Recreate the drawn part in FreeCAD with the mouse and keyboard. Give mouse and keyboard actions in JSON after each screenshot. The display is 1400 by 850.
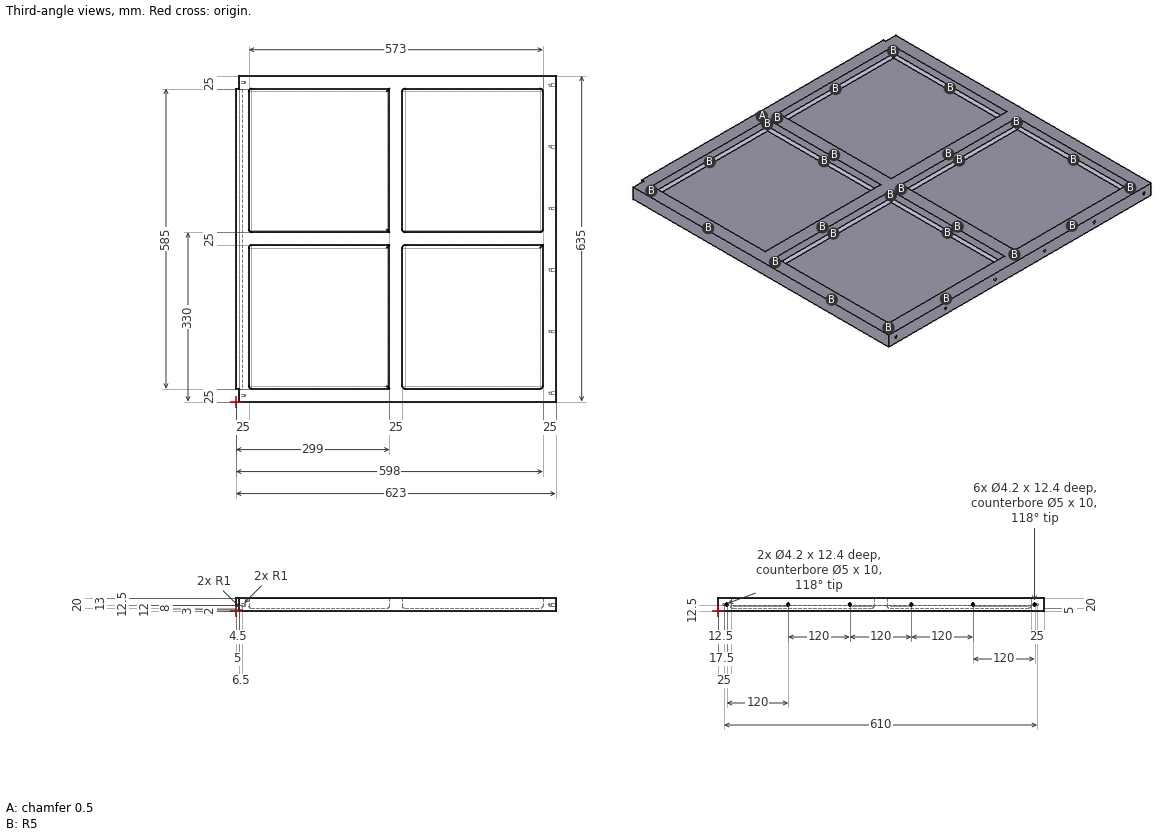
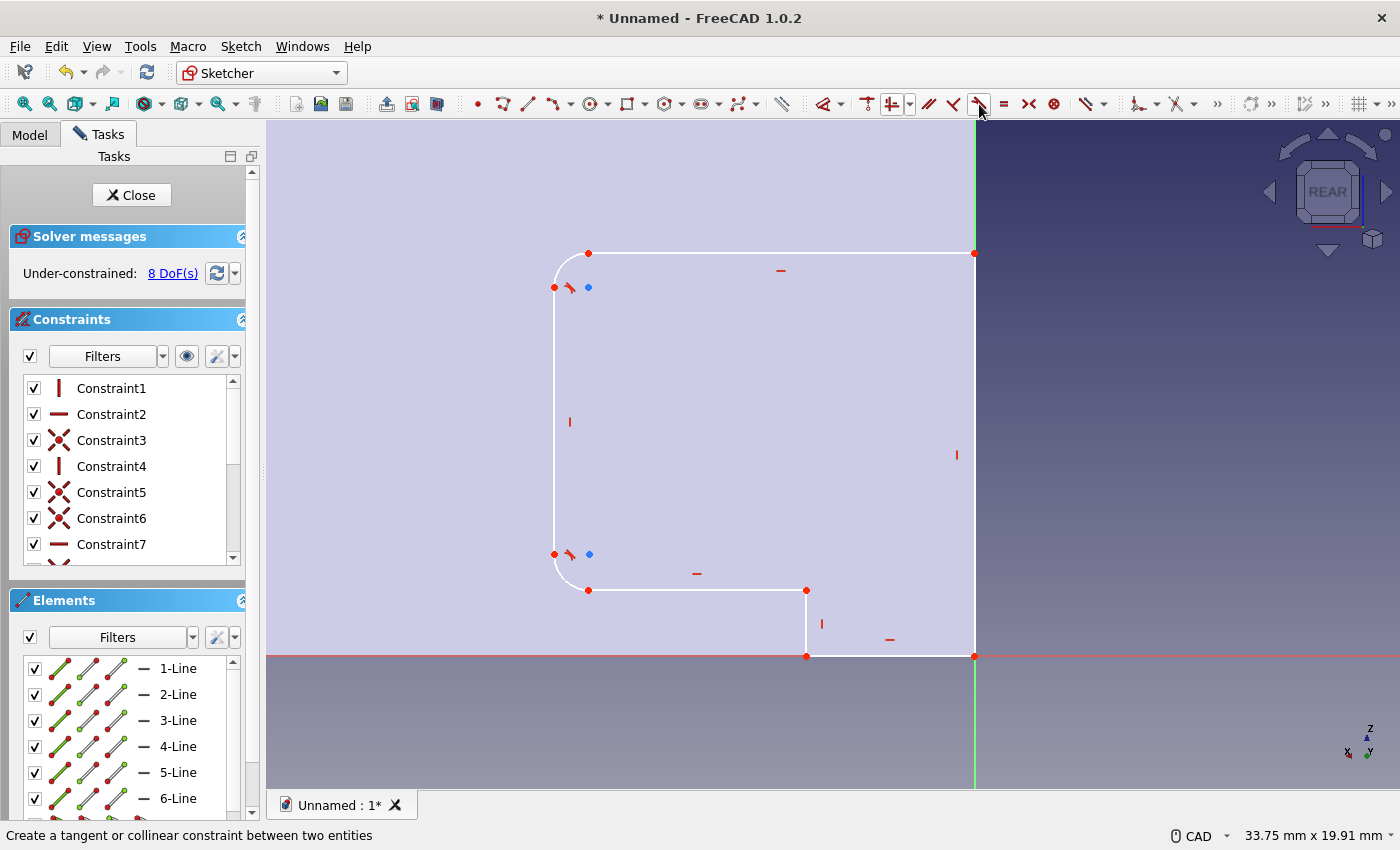
{"action": "left_click", "coordinate": [654, 590]}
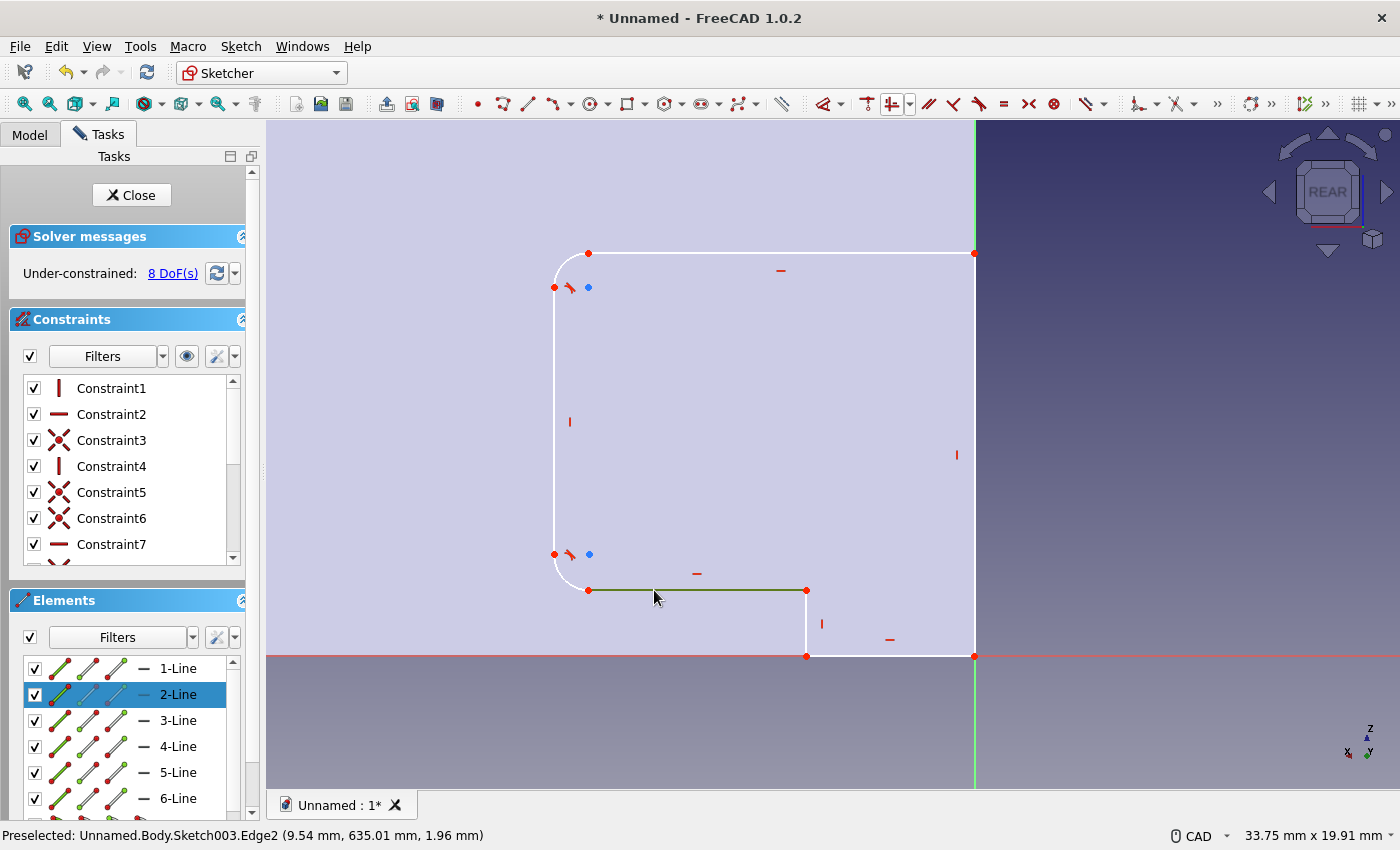
{"action": "left_click", "coordinate": [558, 571]}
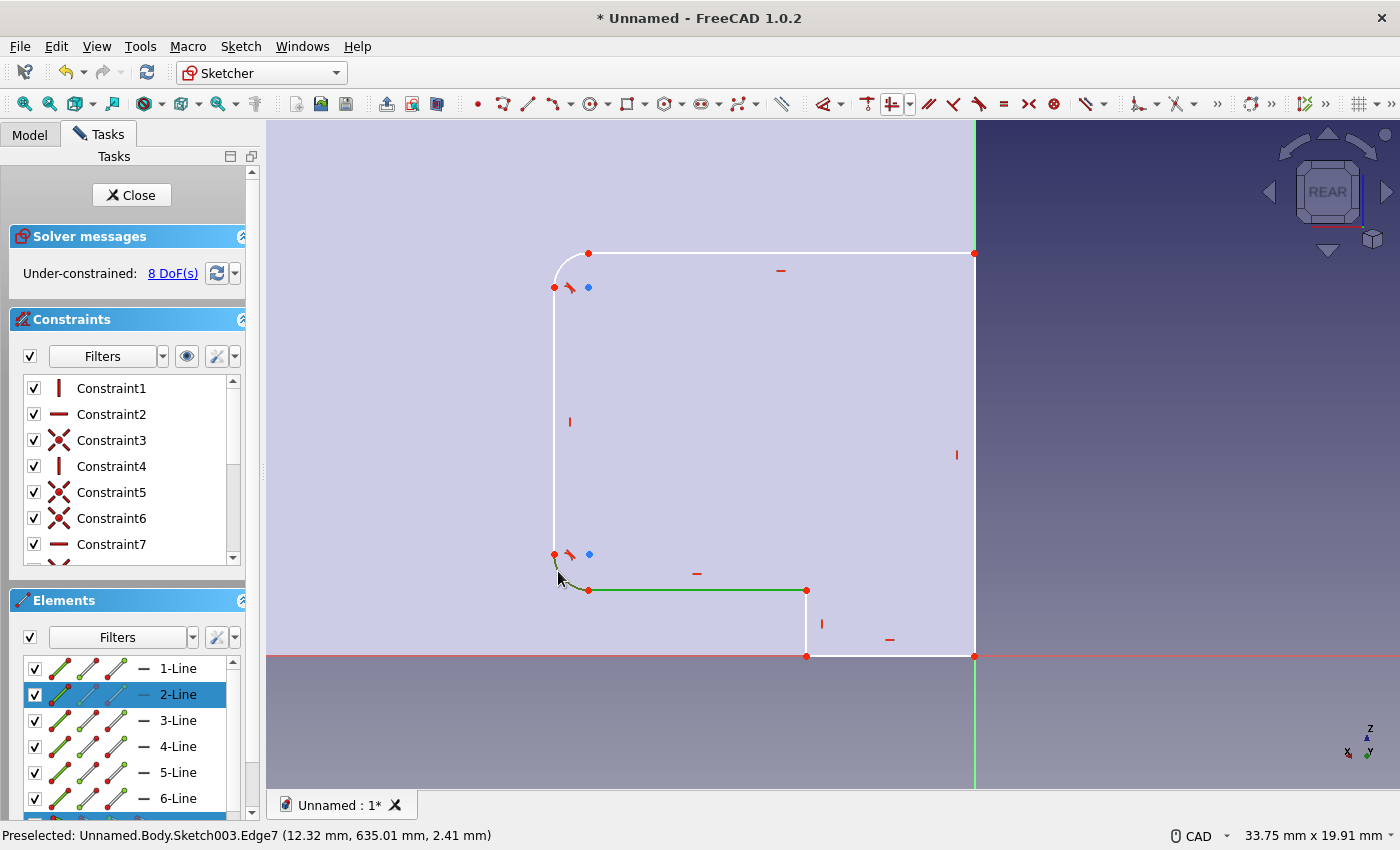
{"action": "left_click", "coordinate": [979, 104]}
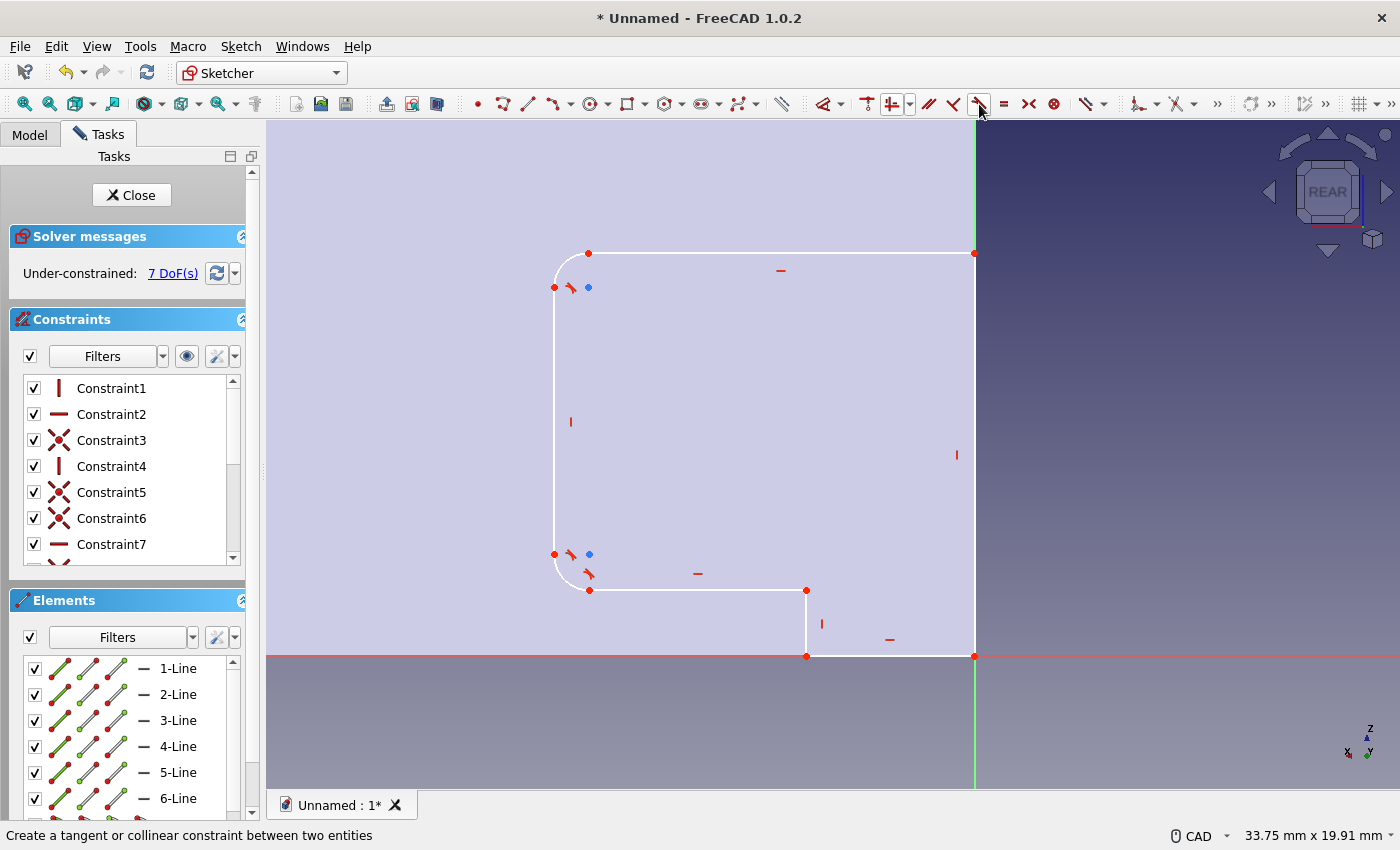
{"action": "left_click", "coordinate": [859, 253]}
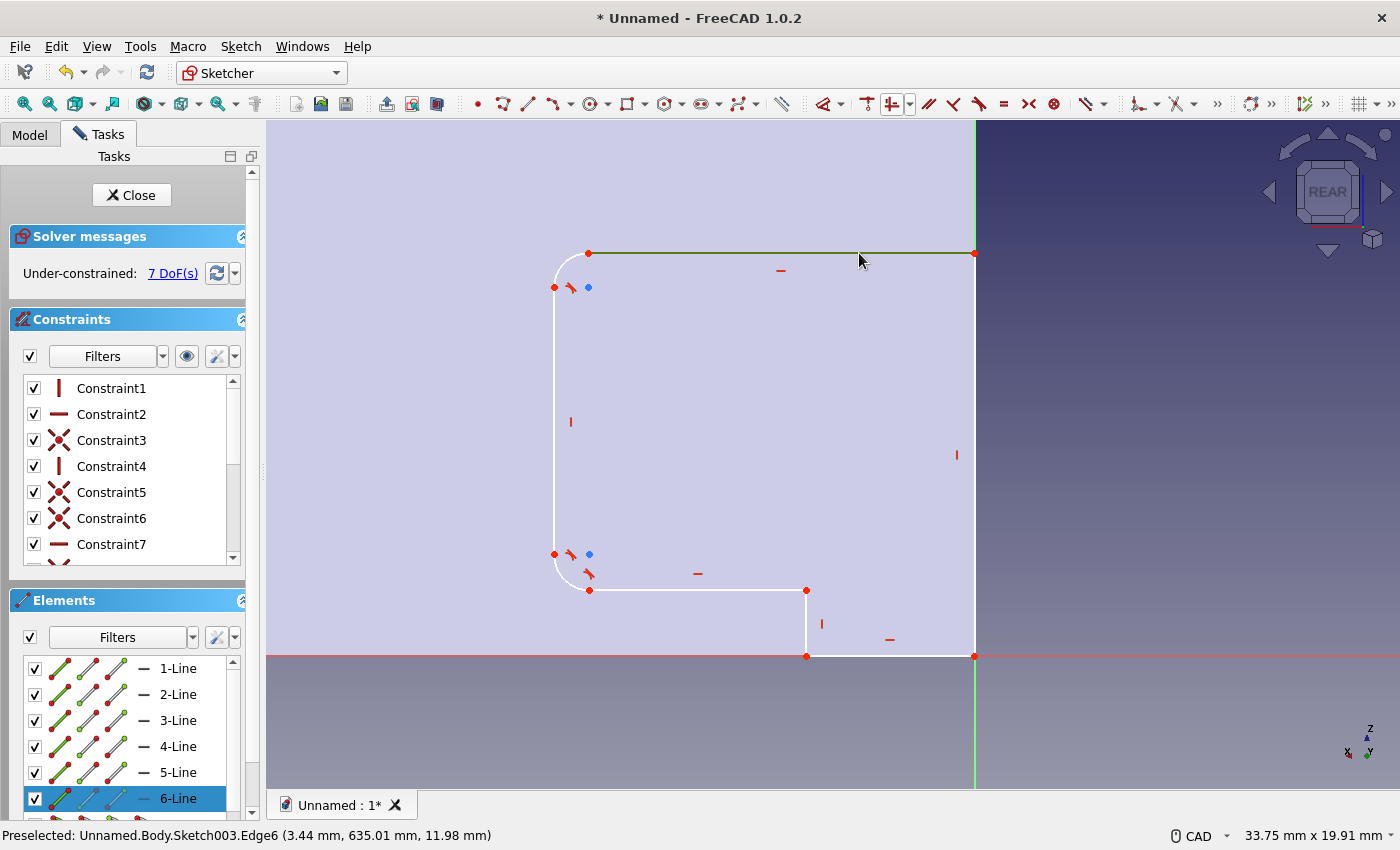
{"action": "left_click", "coordinate": [573, 257]}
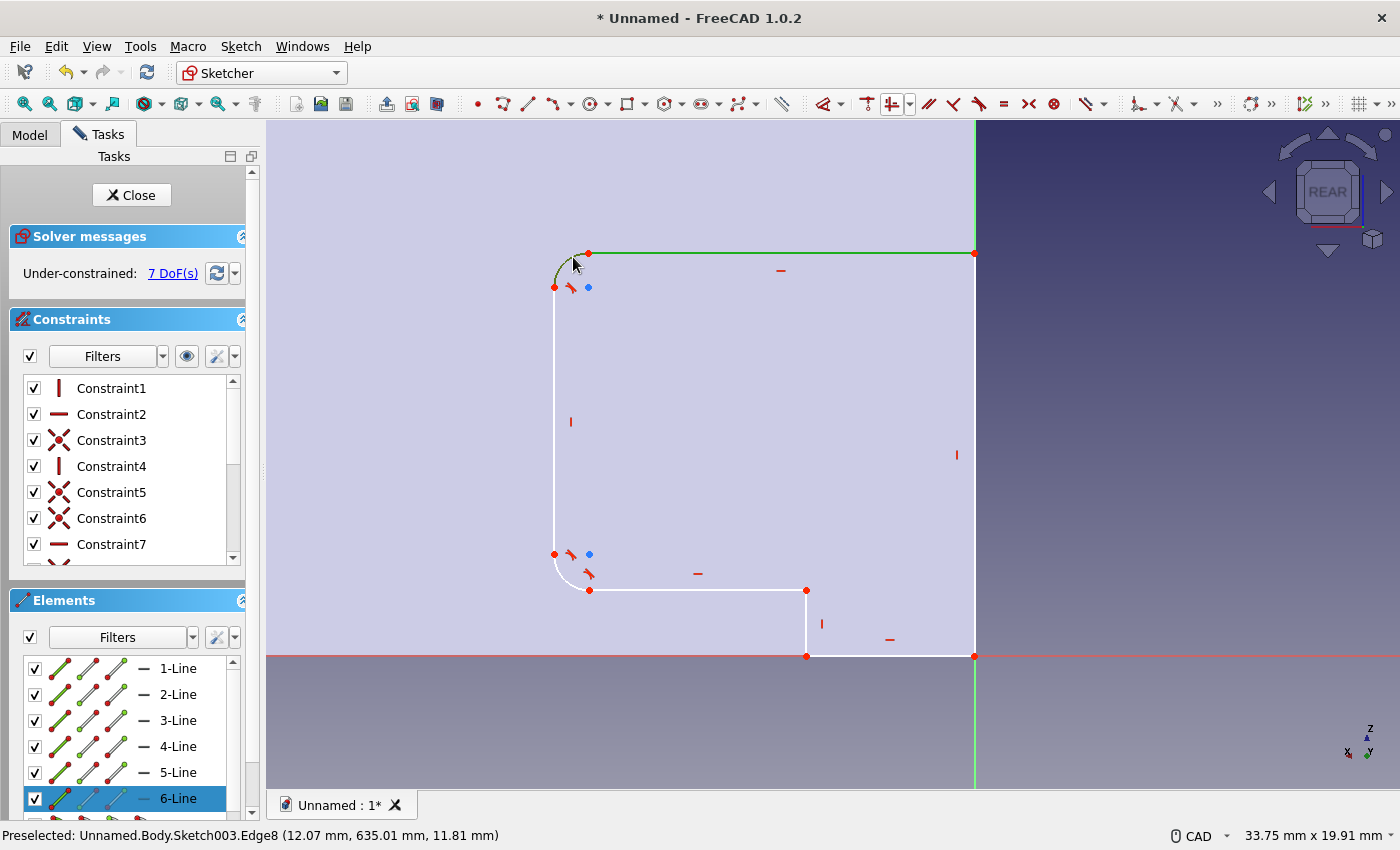
{"action": "left_click", "coordinate": [979, 104]}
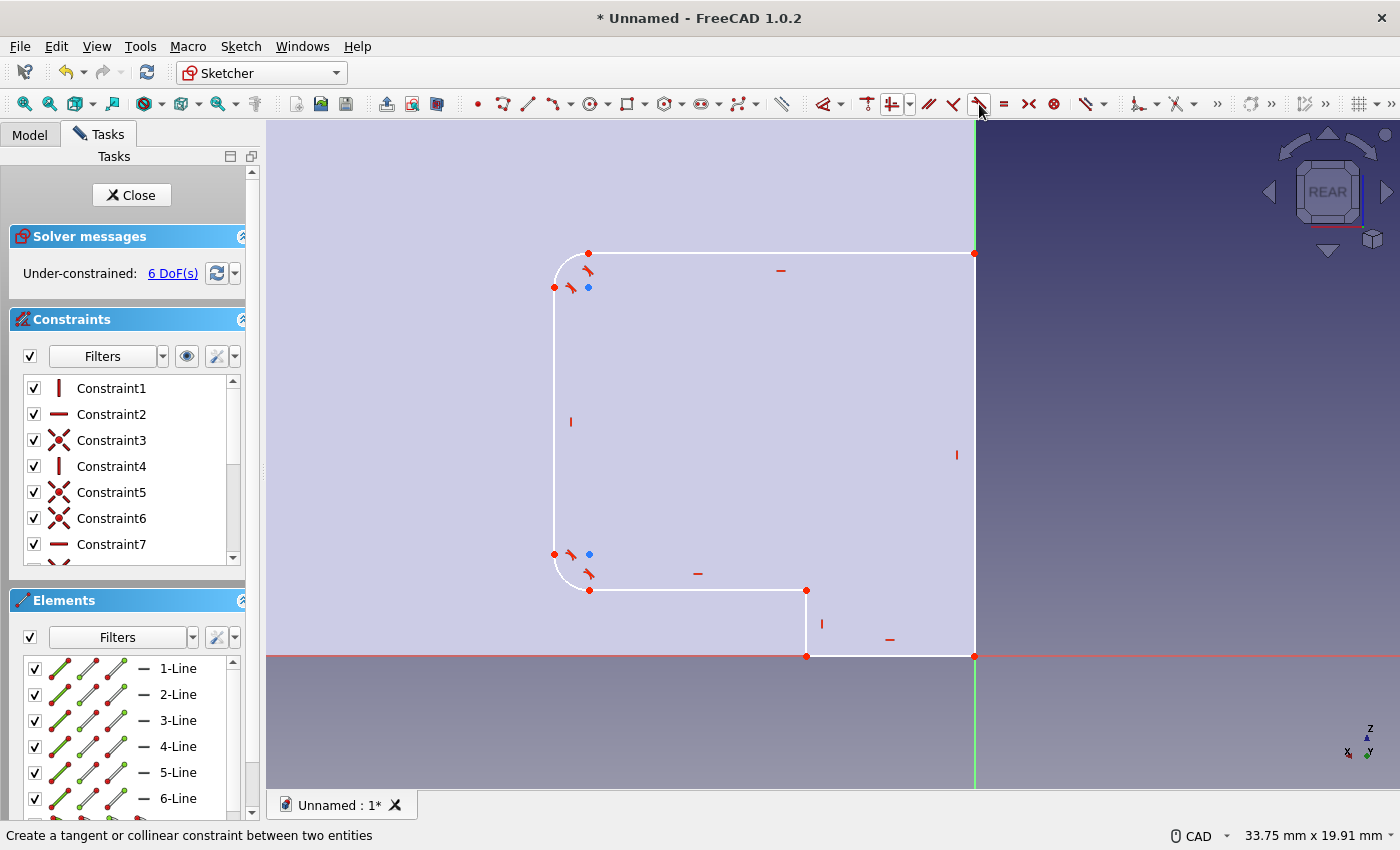
{"action": "left_click", "coordinate": [558, 571]}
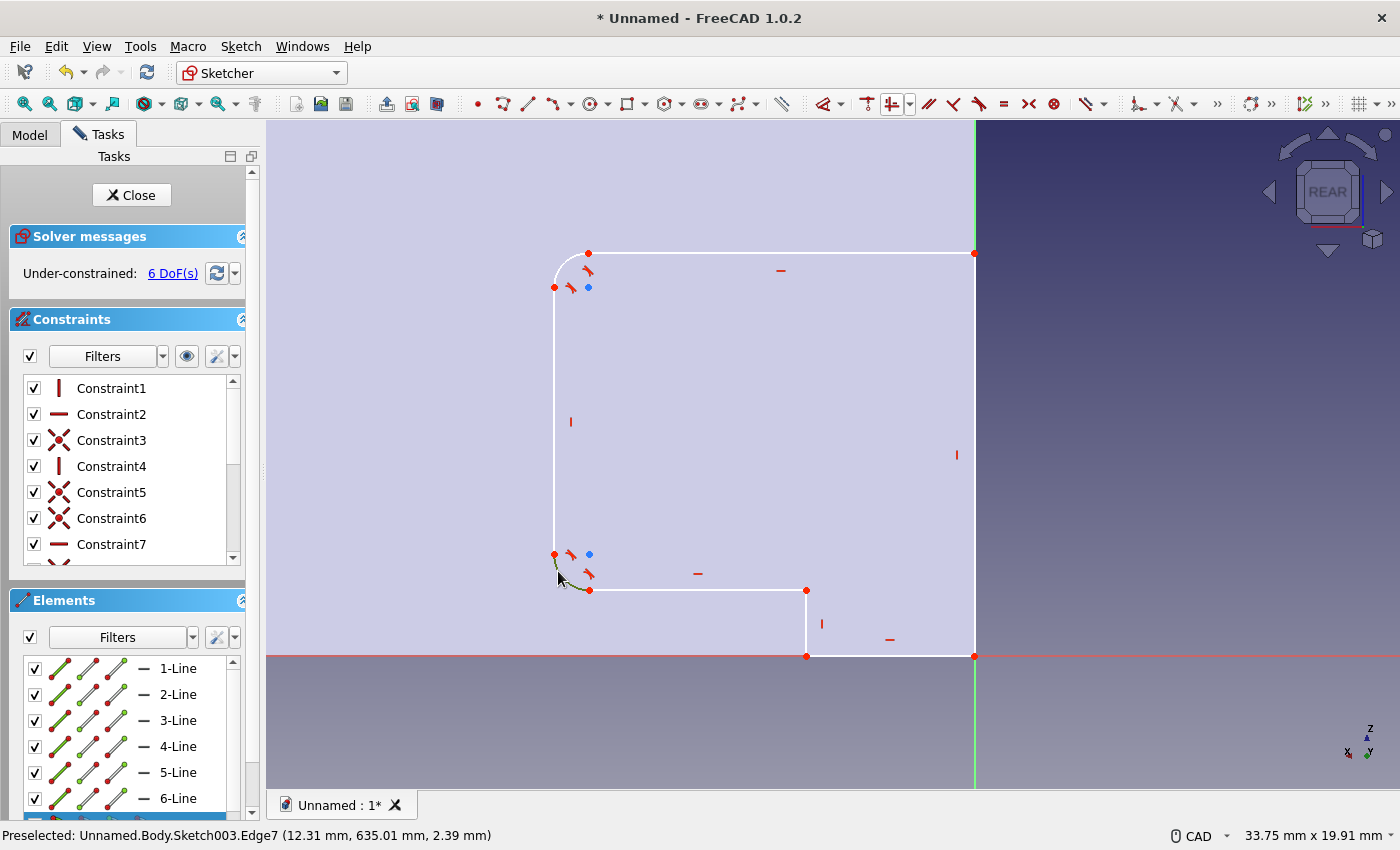
{"action": "left_click", "coordinate": [573, 257]}